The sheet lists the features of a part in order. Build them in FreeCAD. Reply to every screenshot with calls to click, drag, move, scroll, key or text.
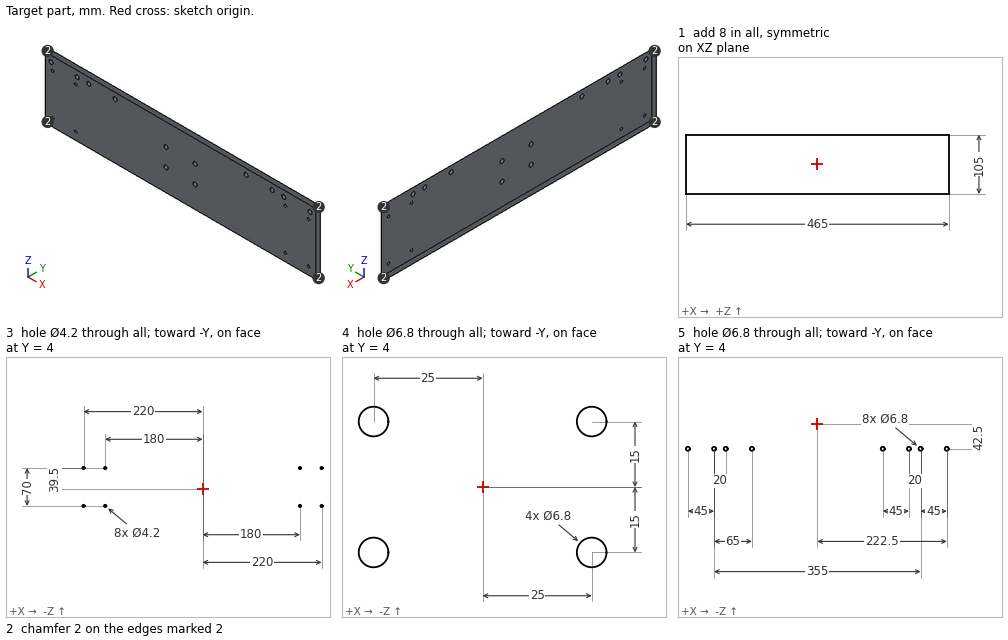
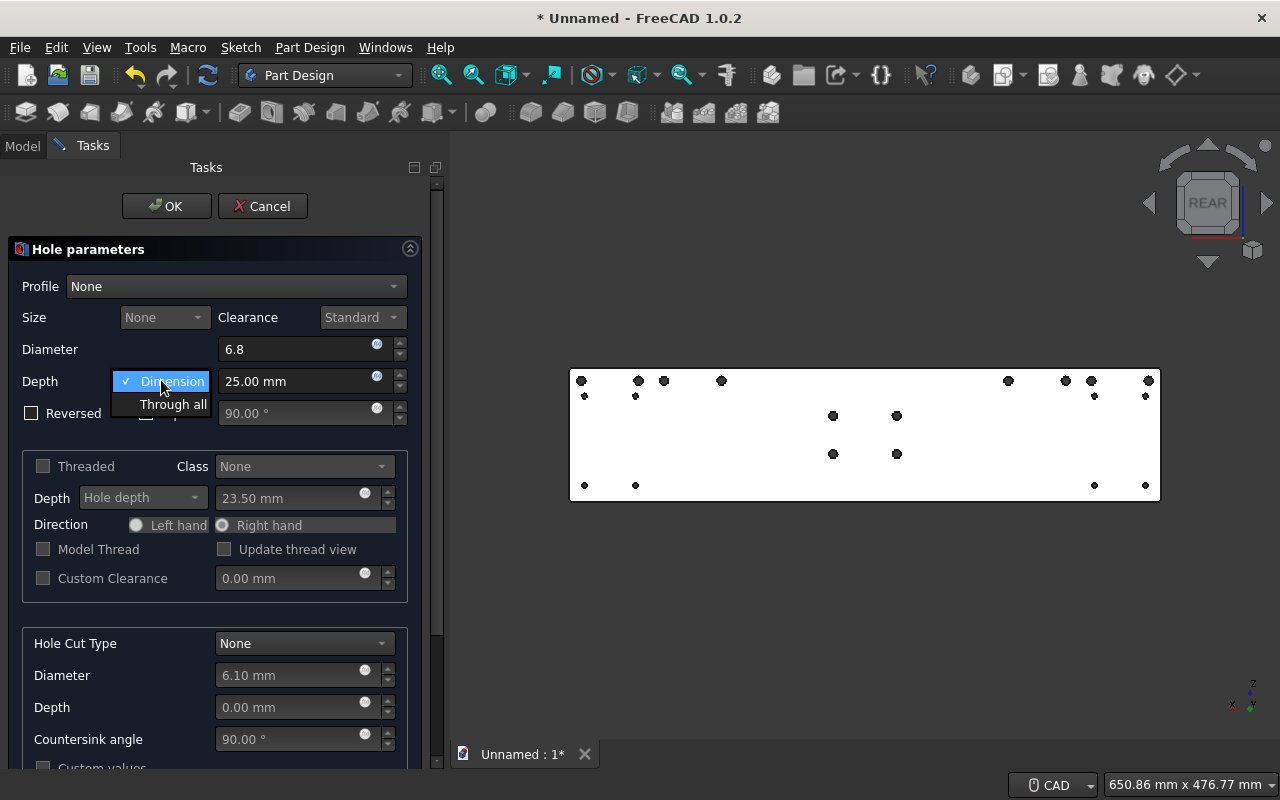
click(160, 404)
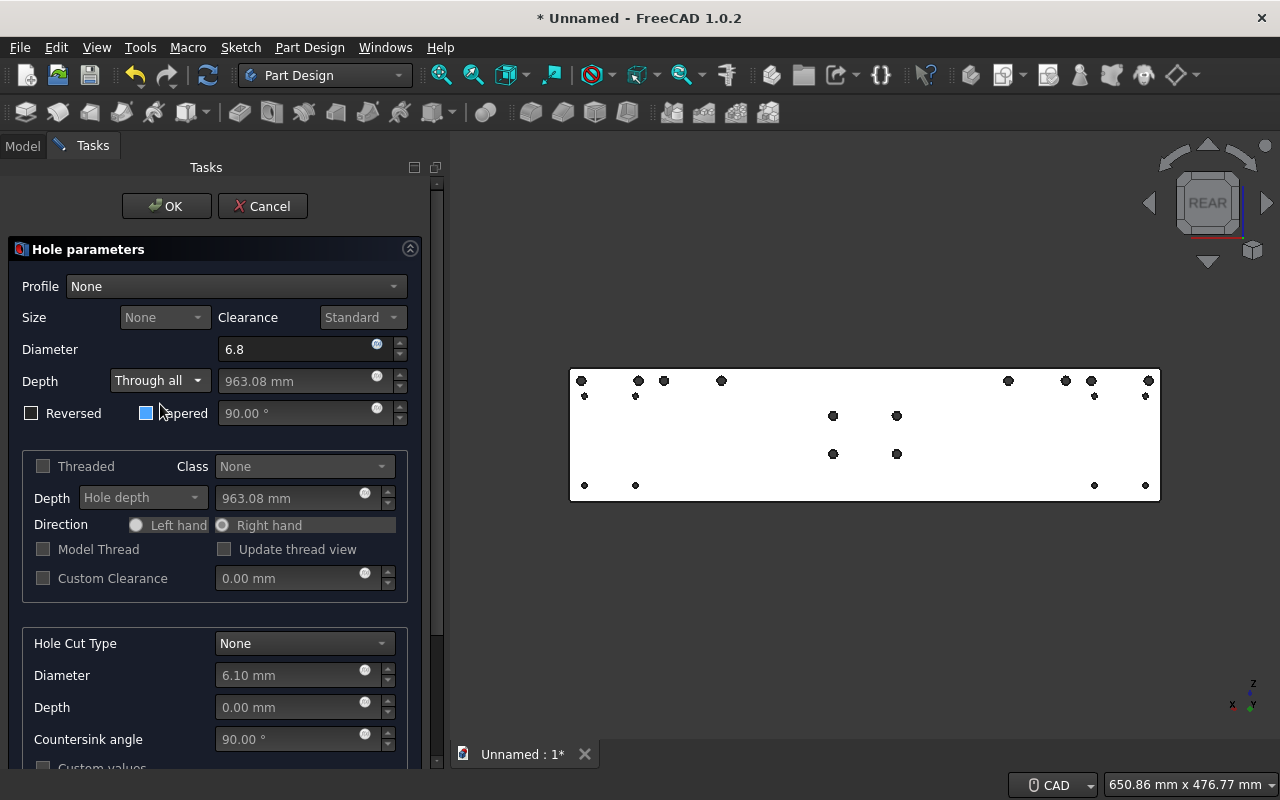
click(167, 206)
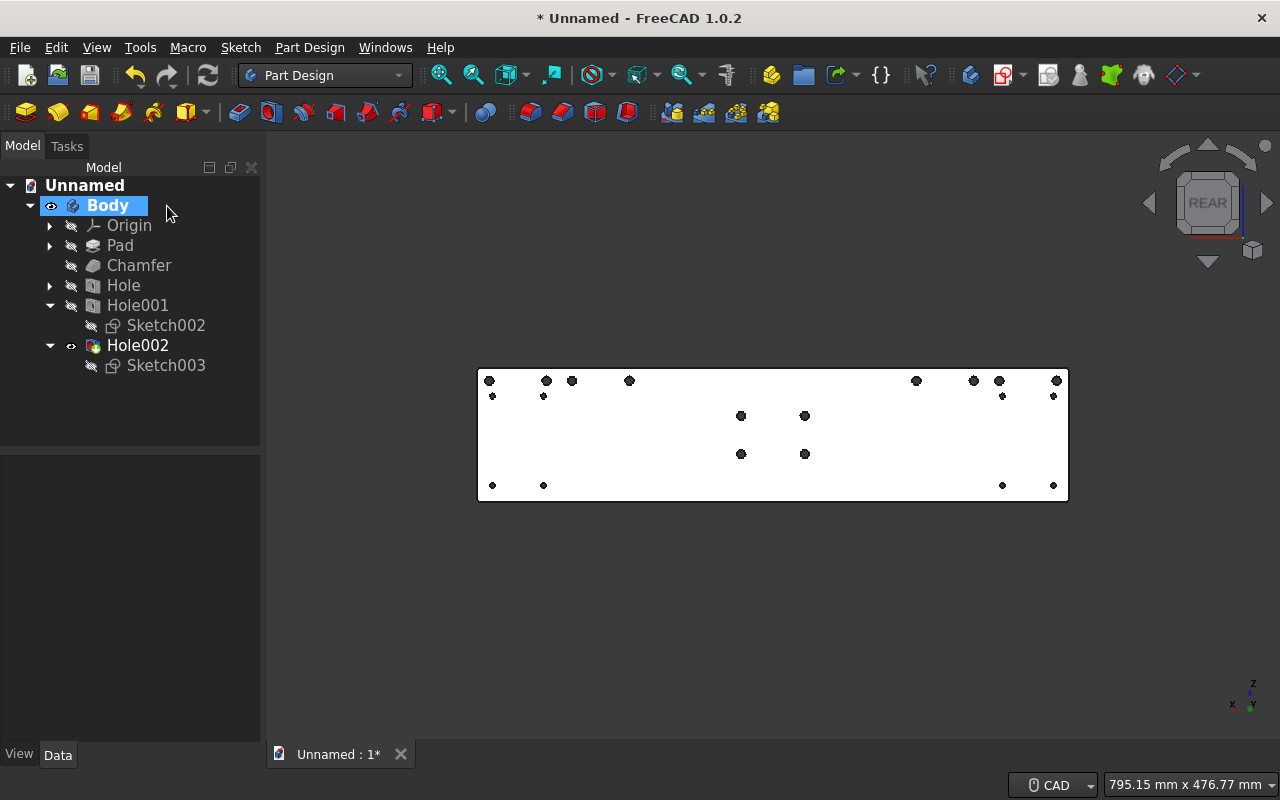
key(0)